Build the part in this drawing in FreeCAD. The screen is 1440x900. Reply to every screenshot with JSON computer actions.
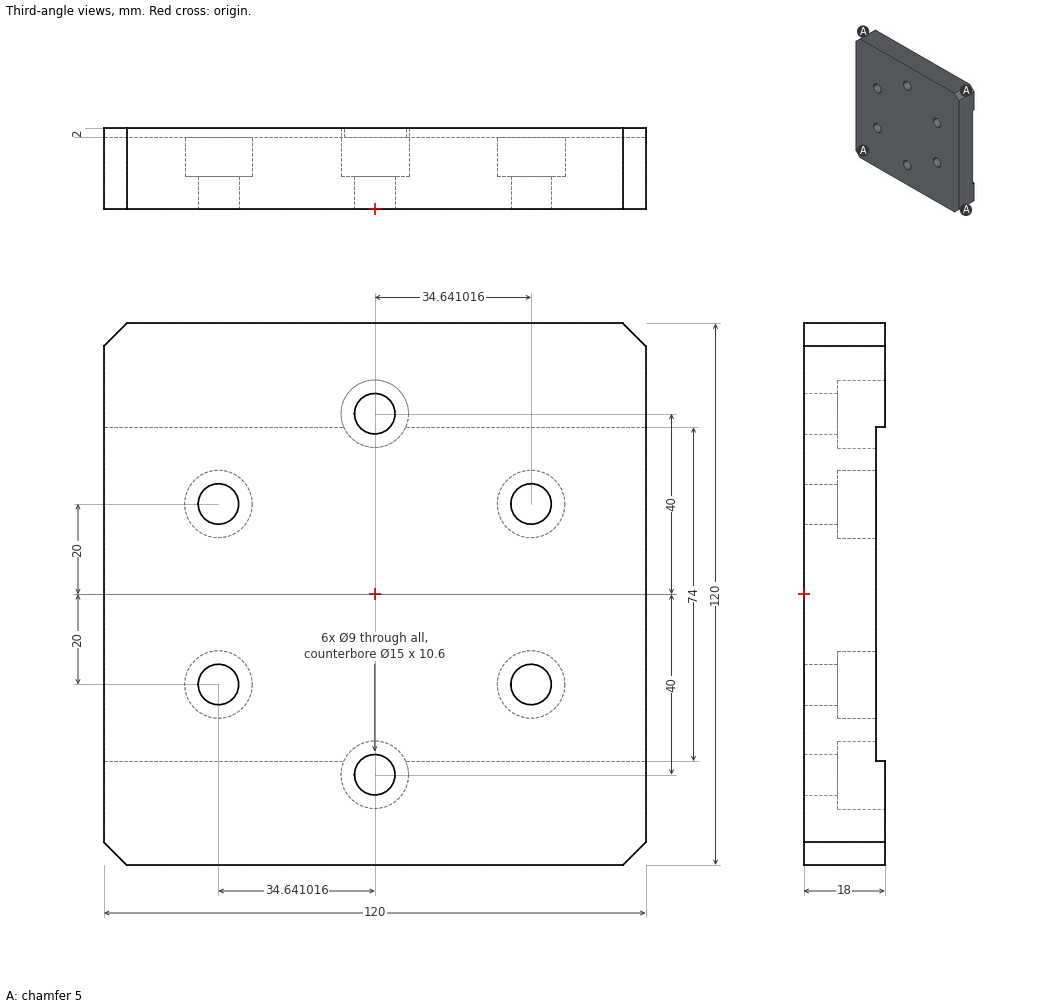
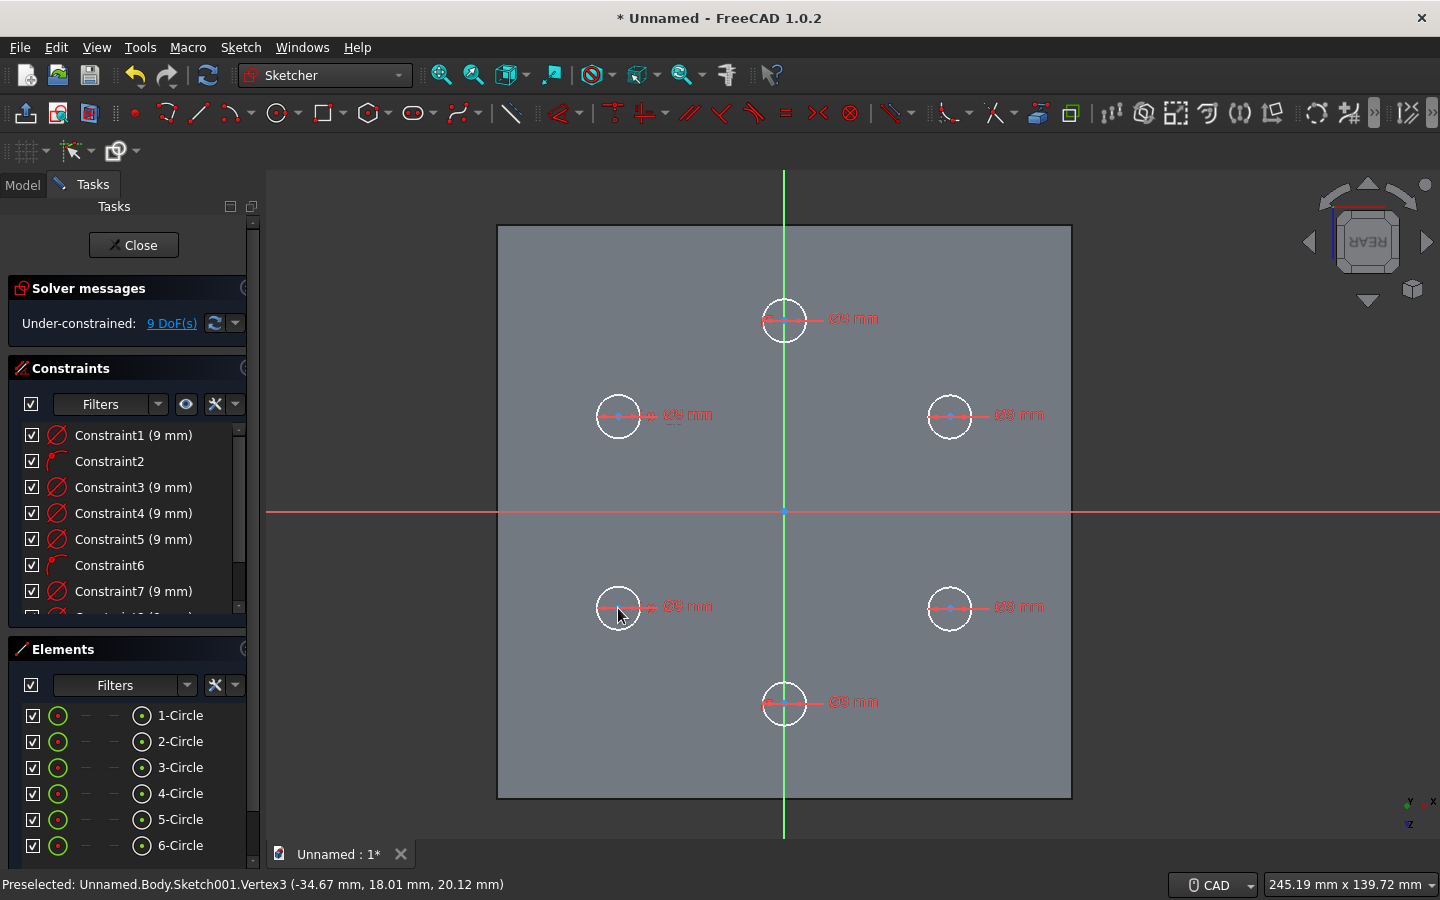
{"action": "left_click", "coordinate": [618, 608]}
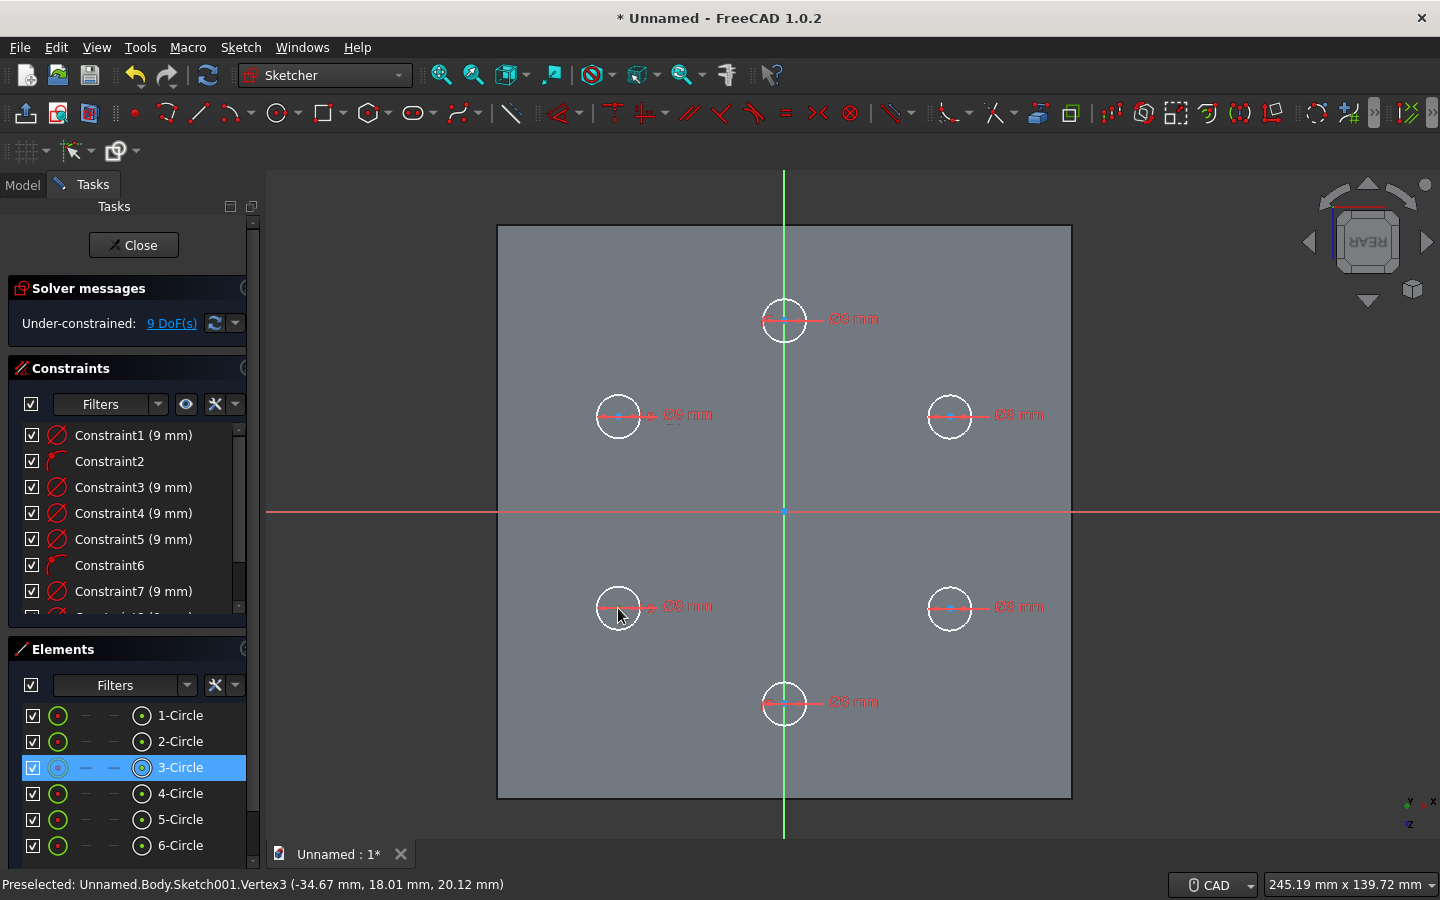
{"action": "left_click", "coordinate": [950, 609]}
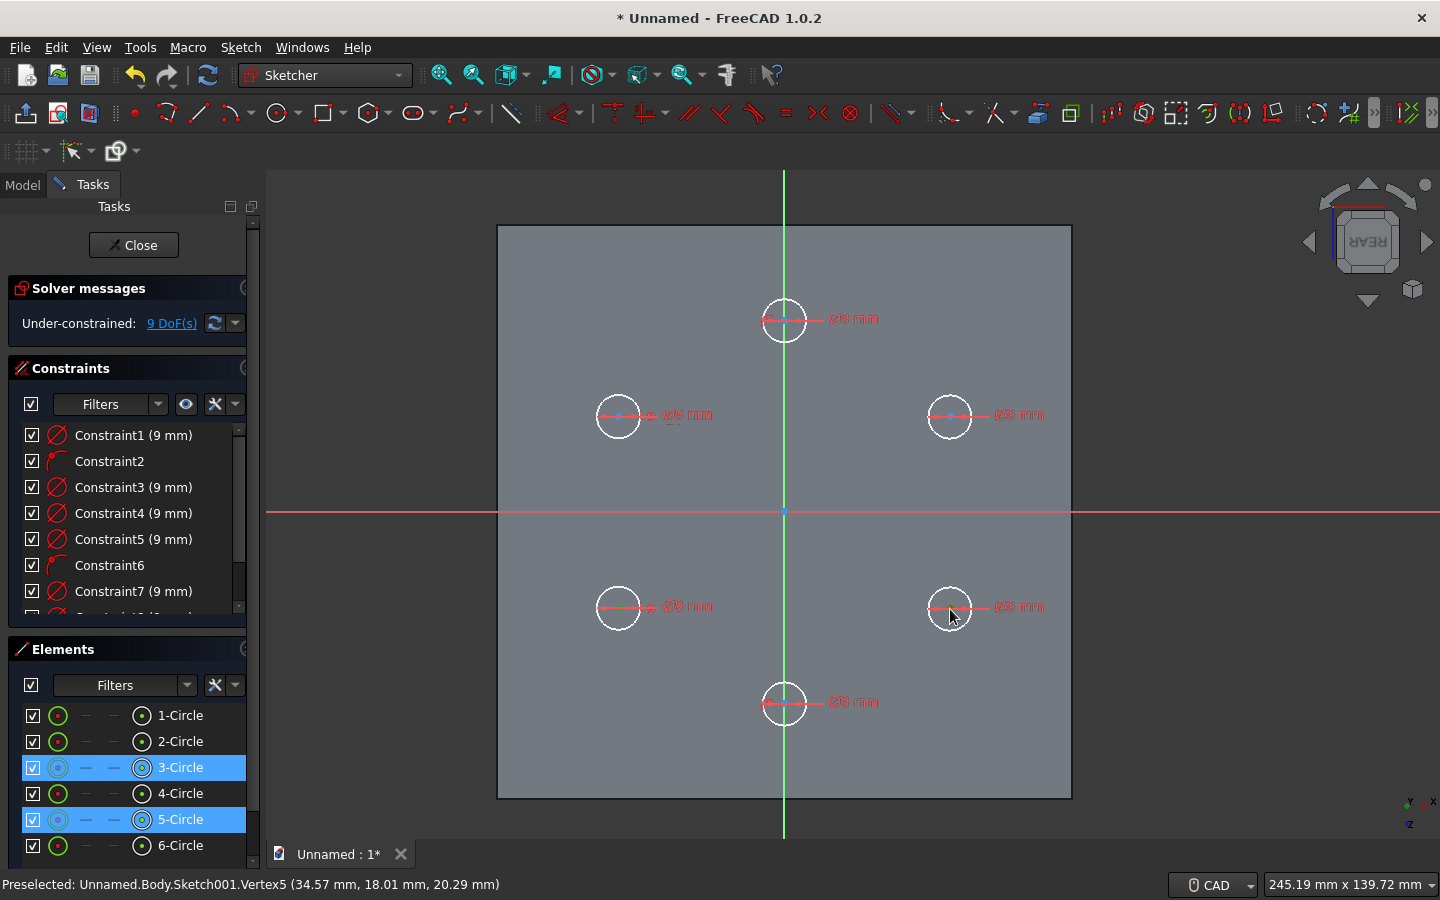
{"action": "key", "text": "h"}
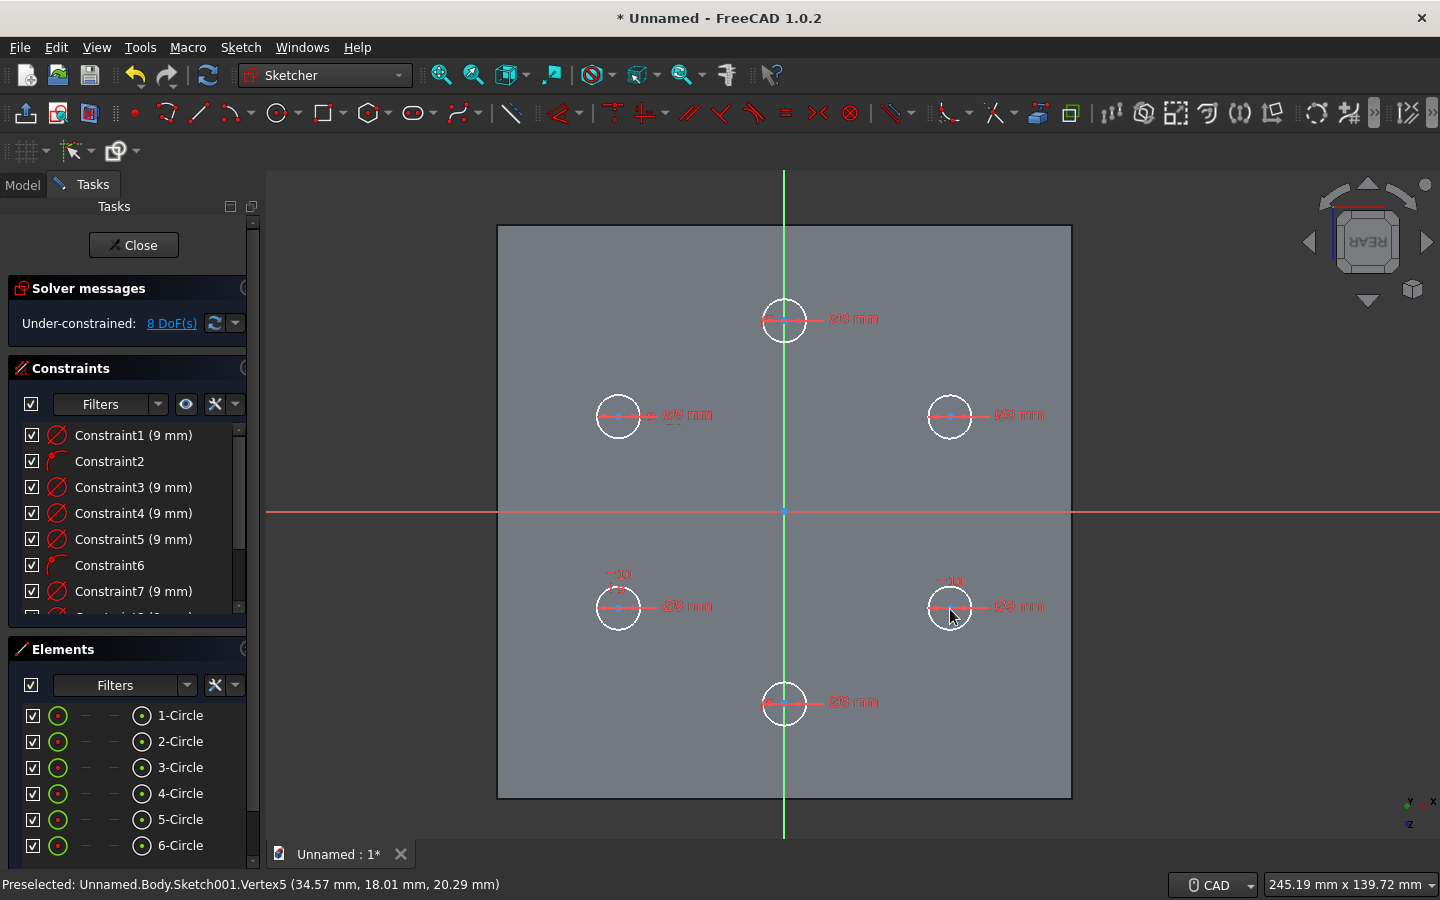
{"action": "left_click", "coordinate": [950, 608]}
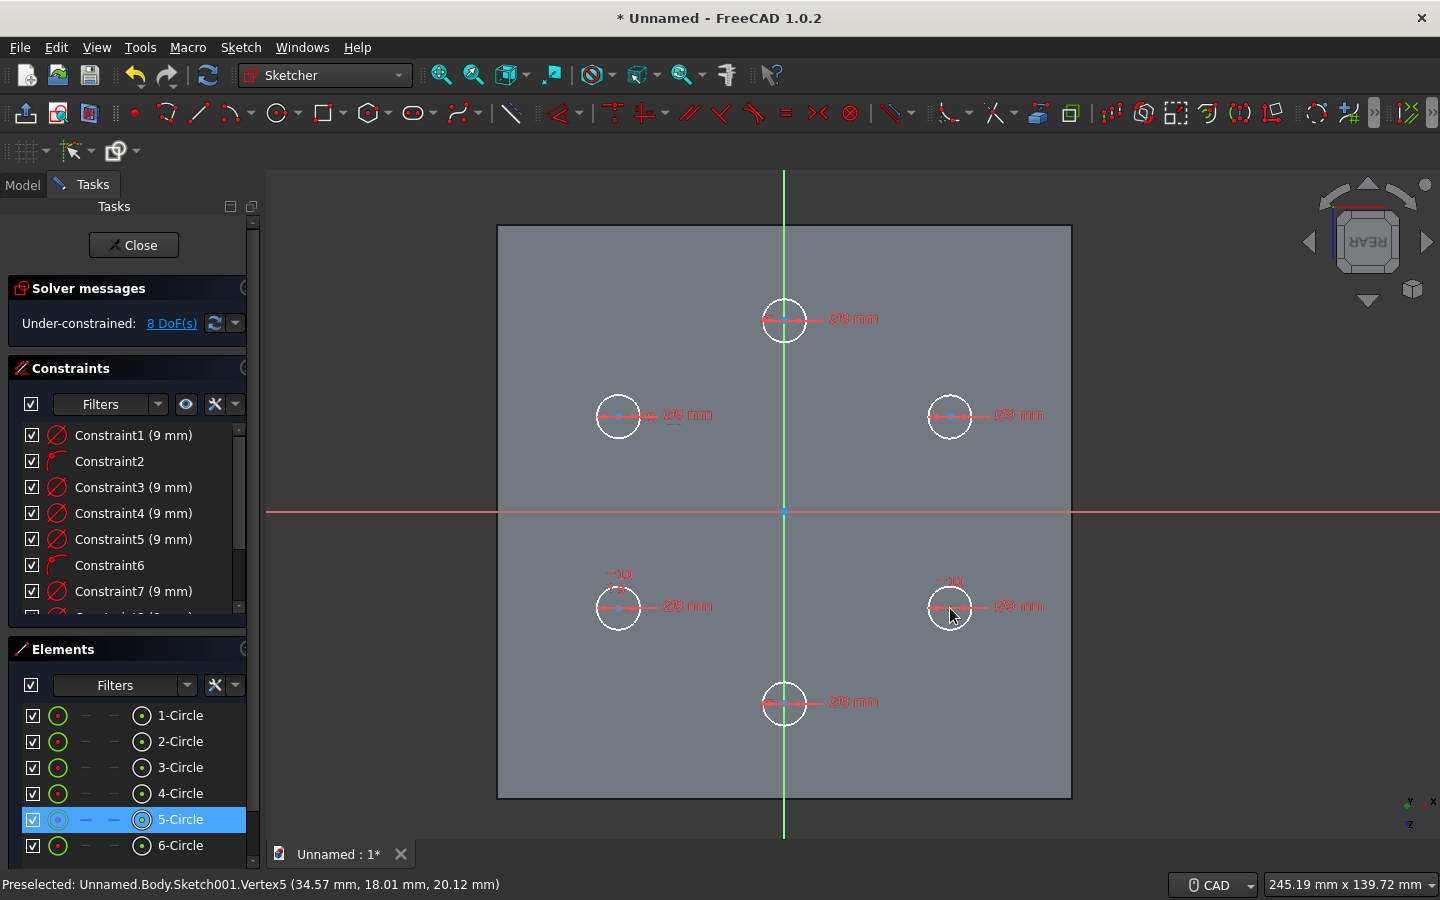
{"action": "left_click", "coordinate": [950, 417]}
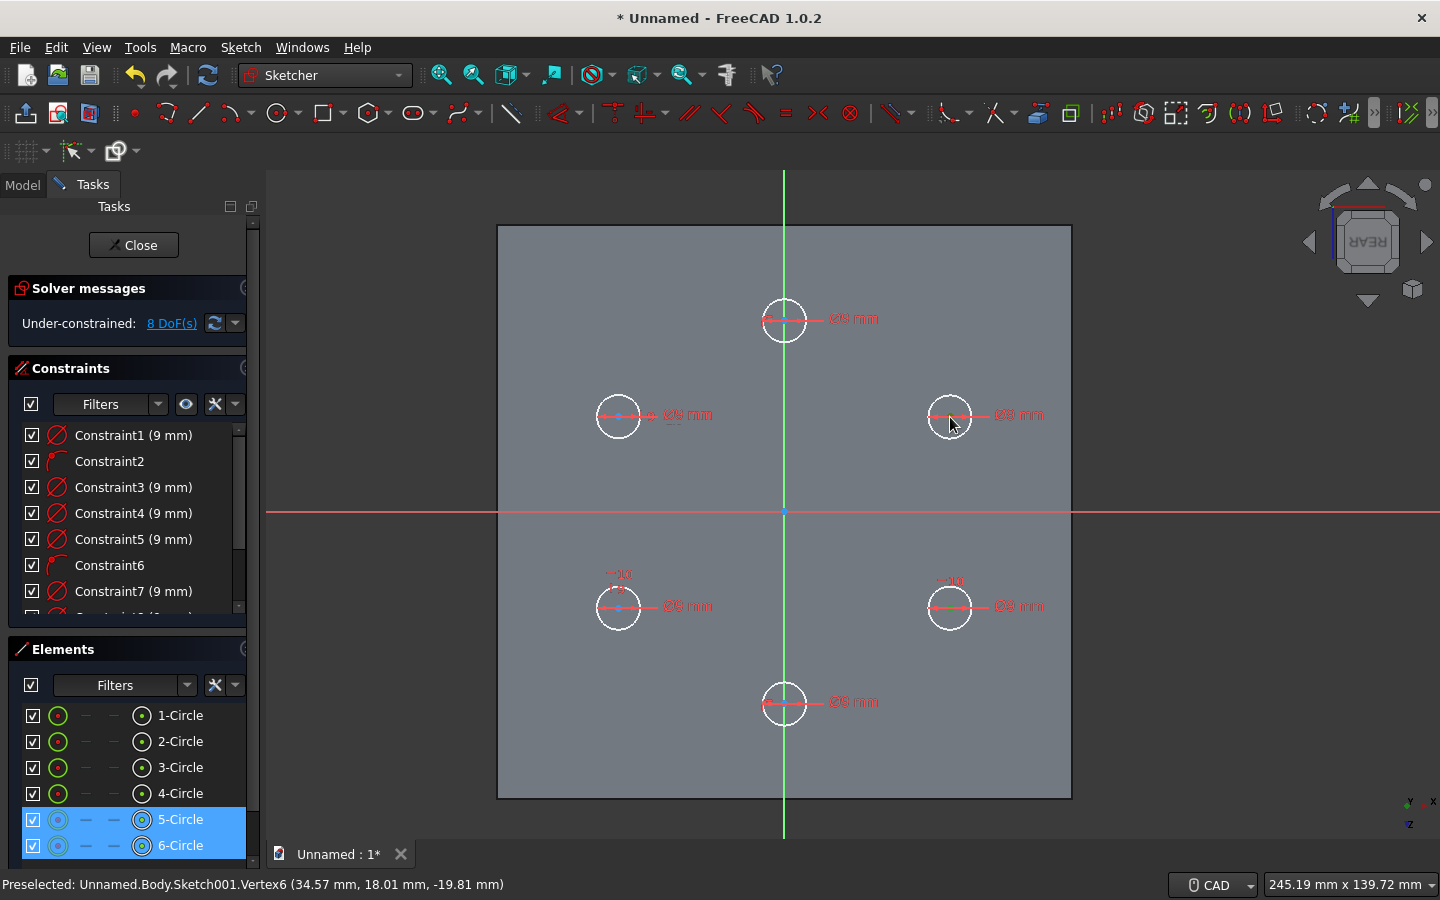
{"action": "left_click", "coordinate": [668, 114]}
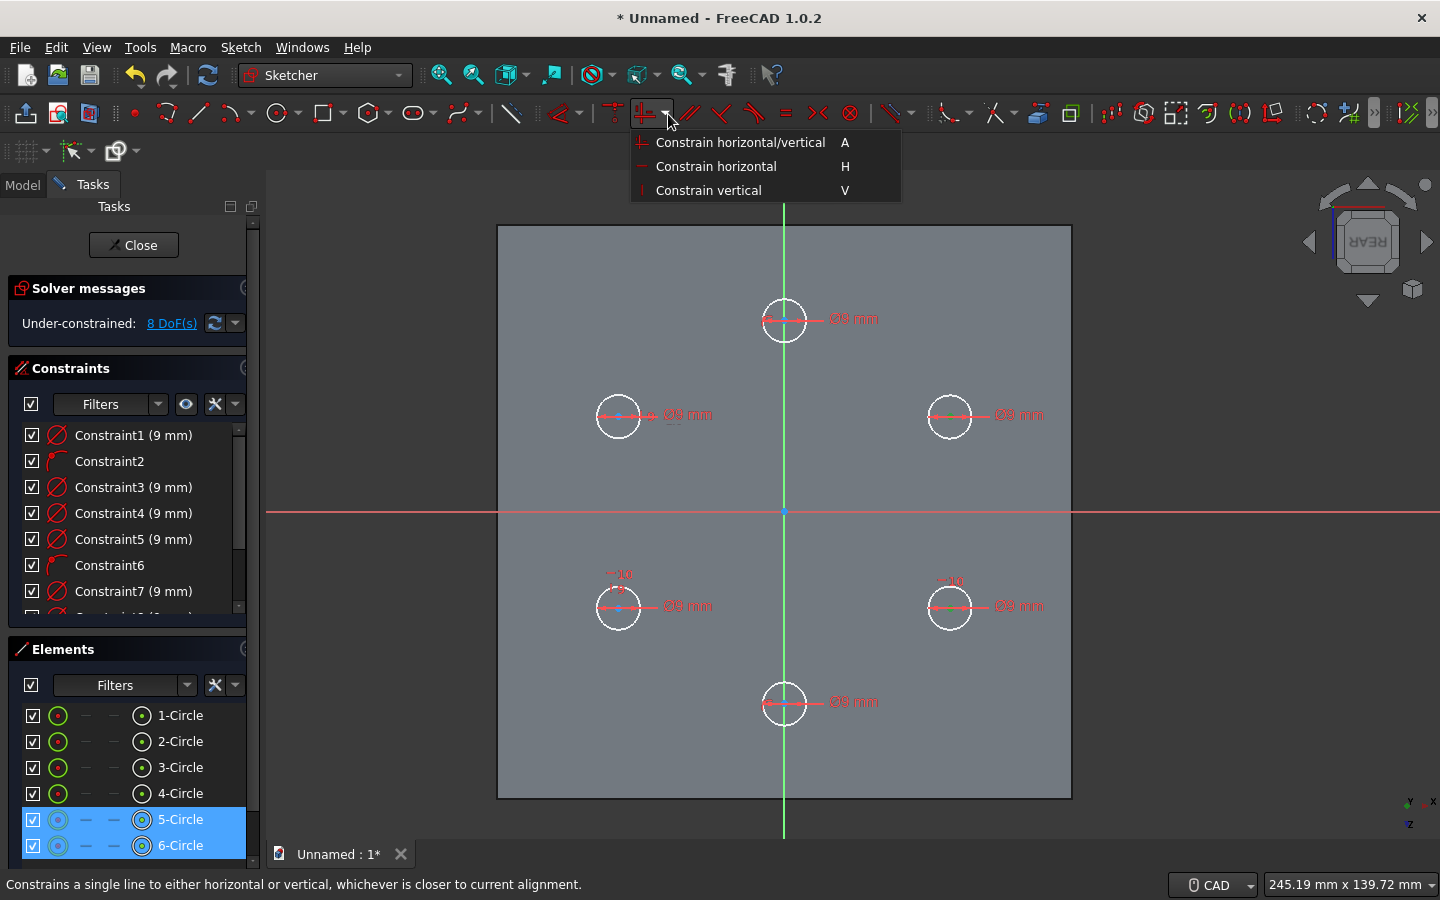
{"action": "left_click", "coordinate": [766, 190]}